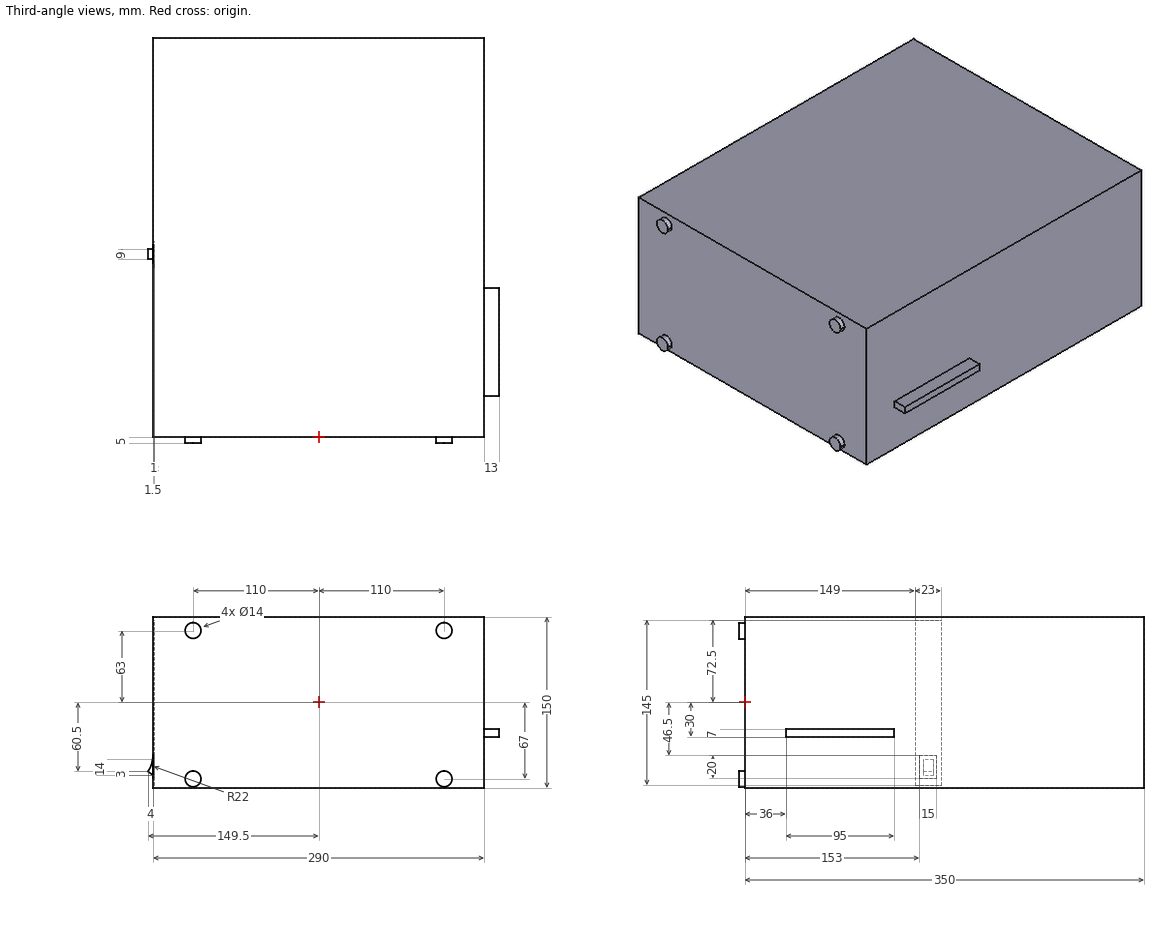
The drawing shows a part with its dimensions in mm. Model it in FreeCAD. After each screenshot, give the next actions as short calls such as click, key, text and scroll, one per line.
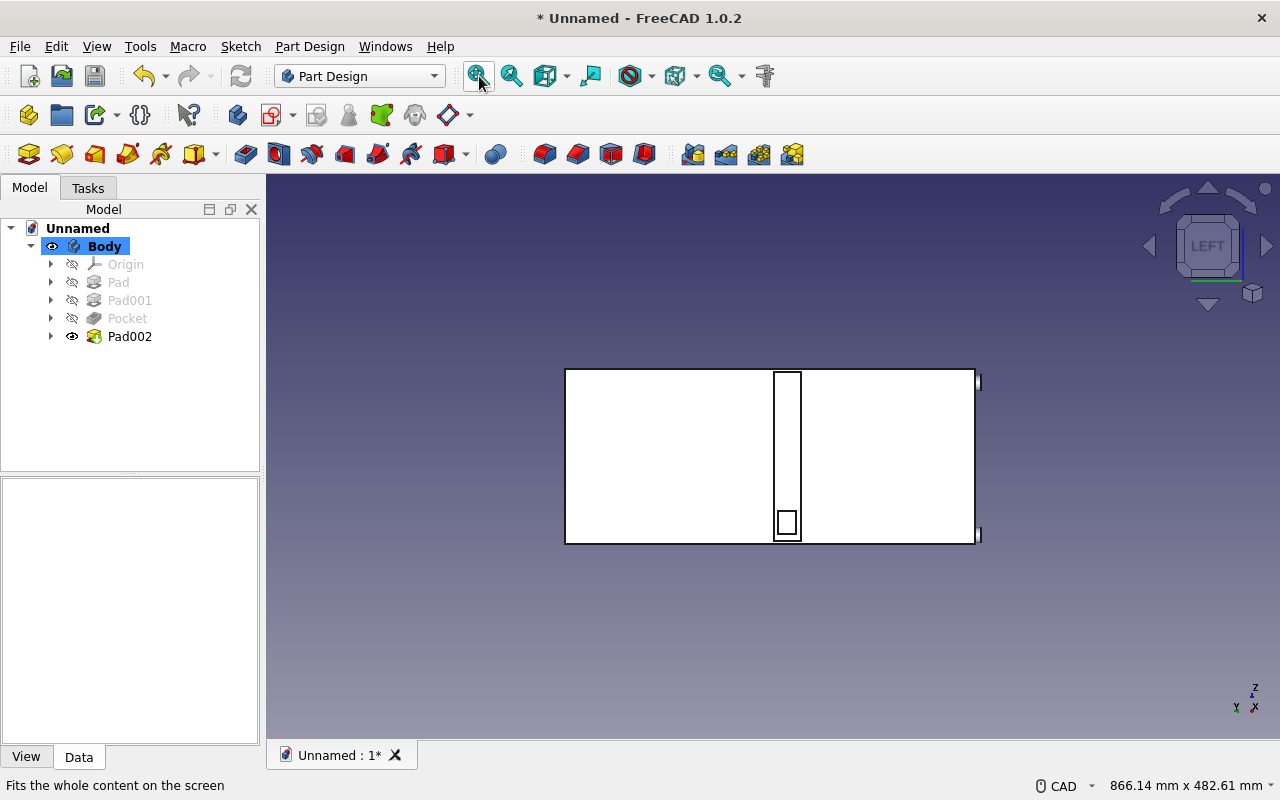
click(51, 264)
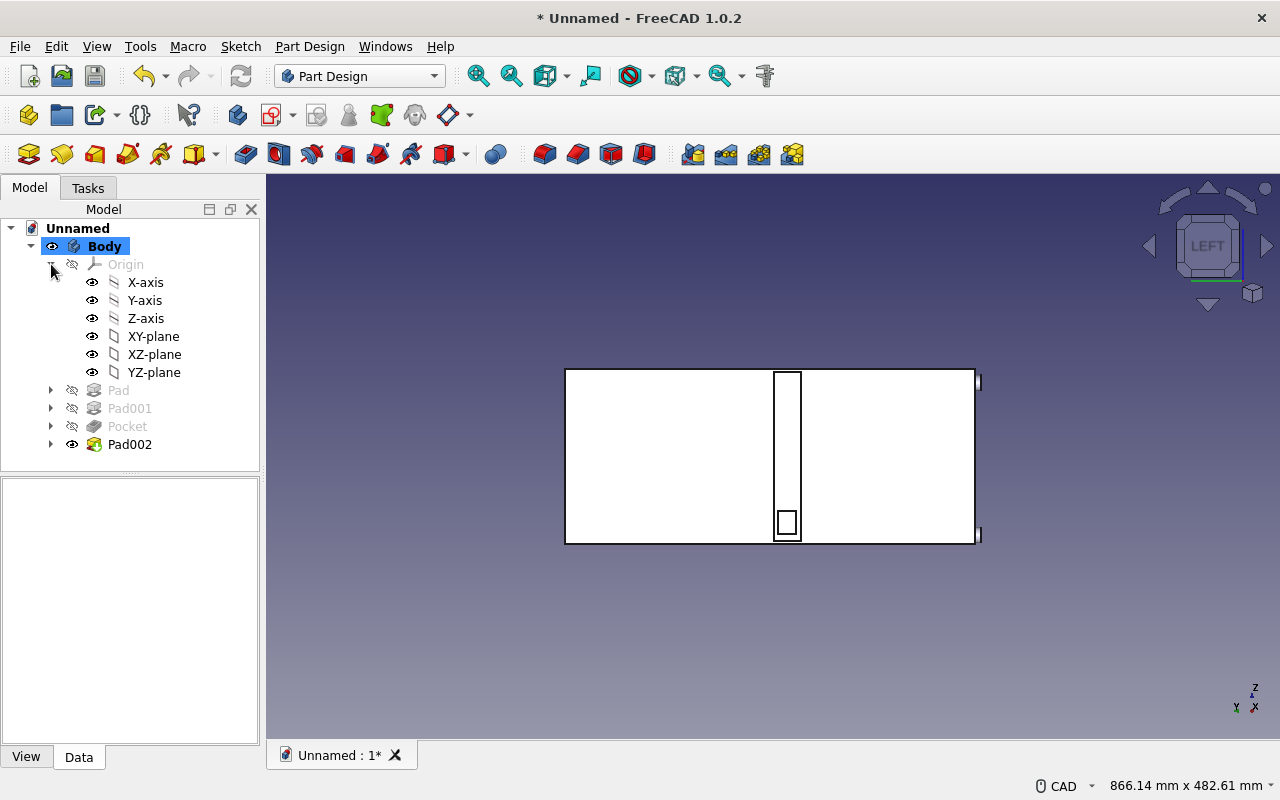
click(137, 354)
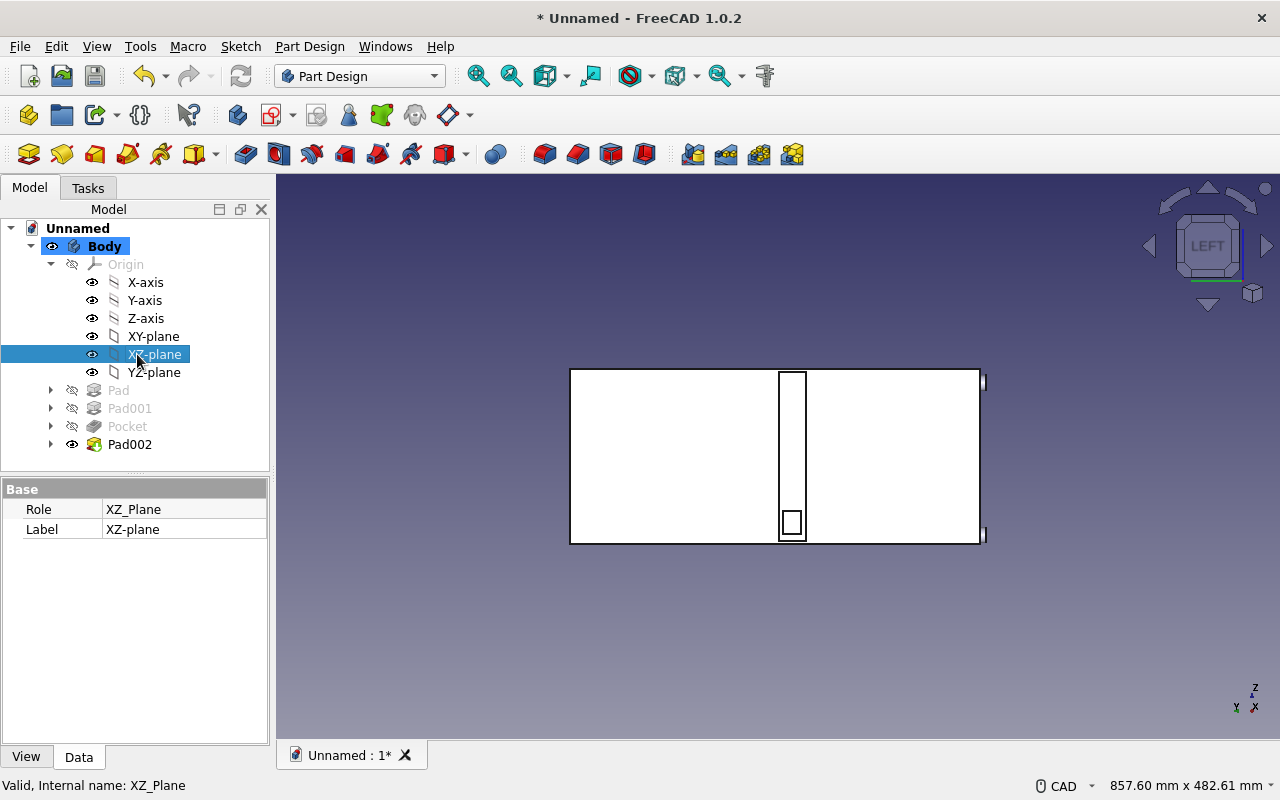
click(448, 116)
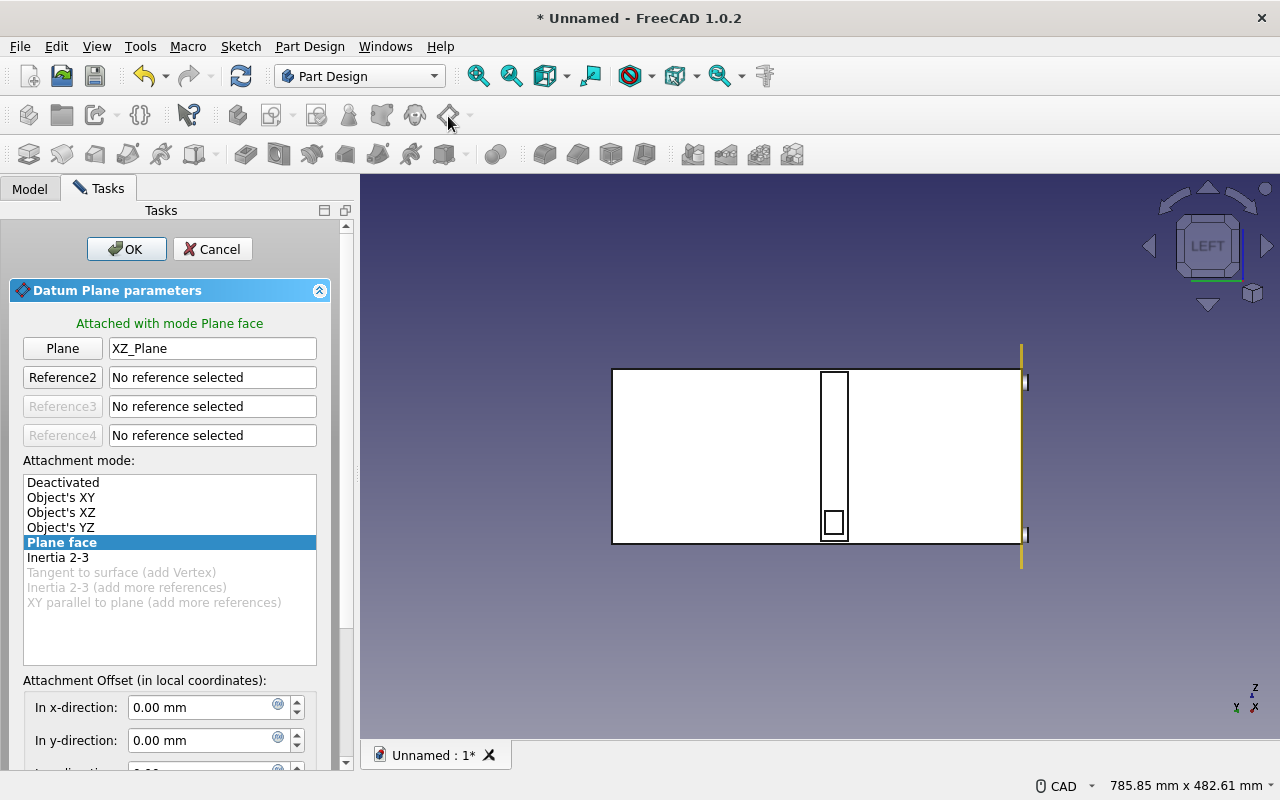
scroll(346, 495, down, 2)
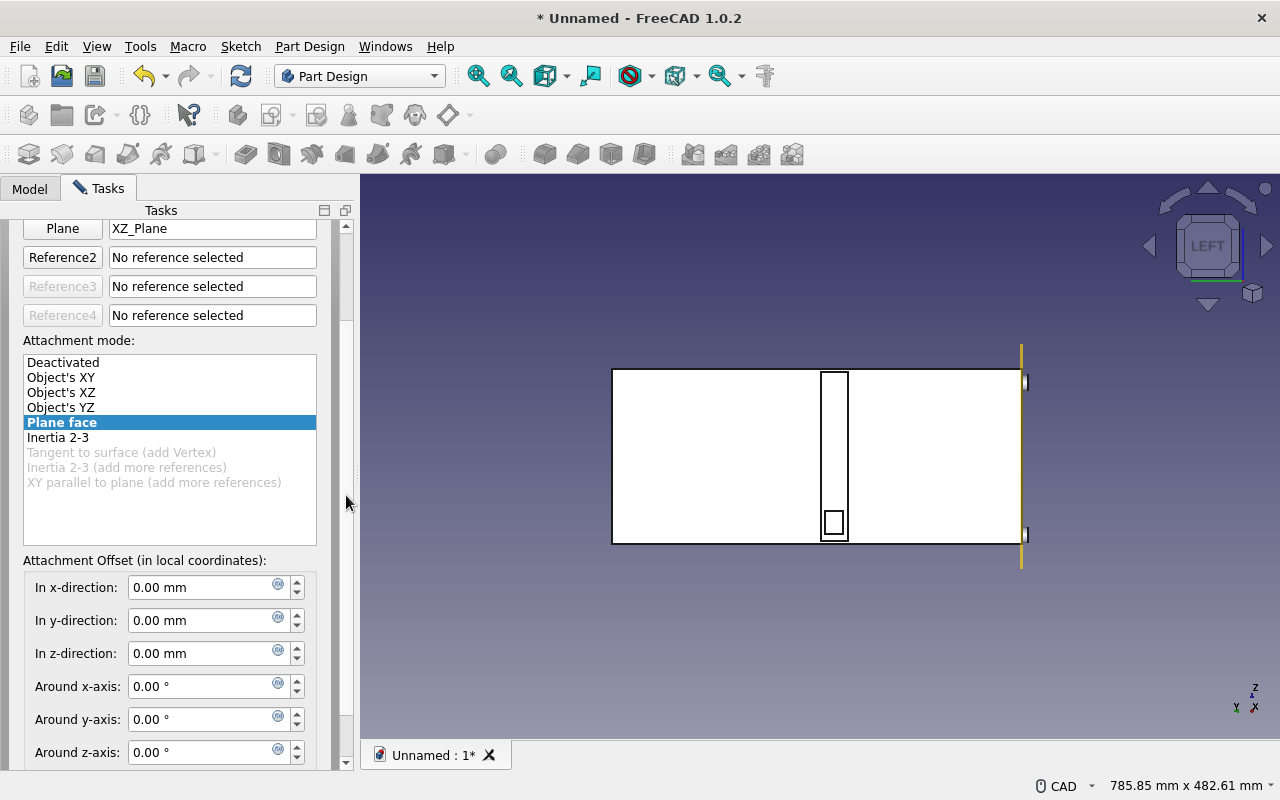
triple_click(210, 654)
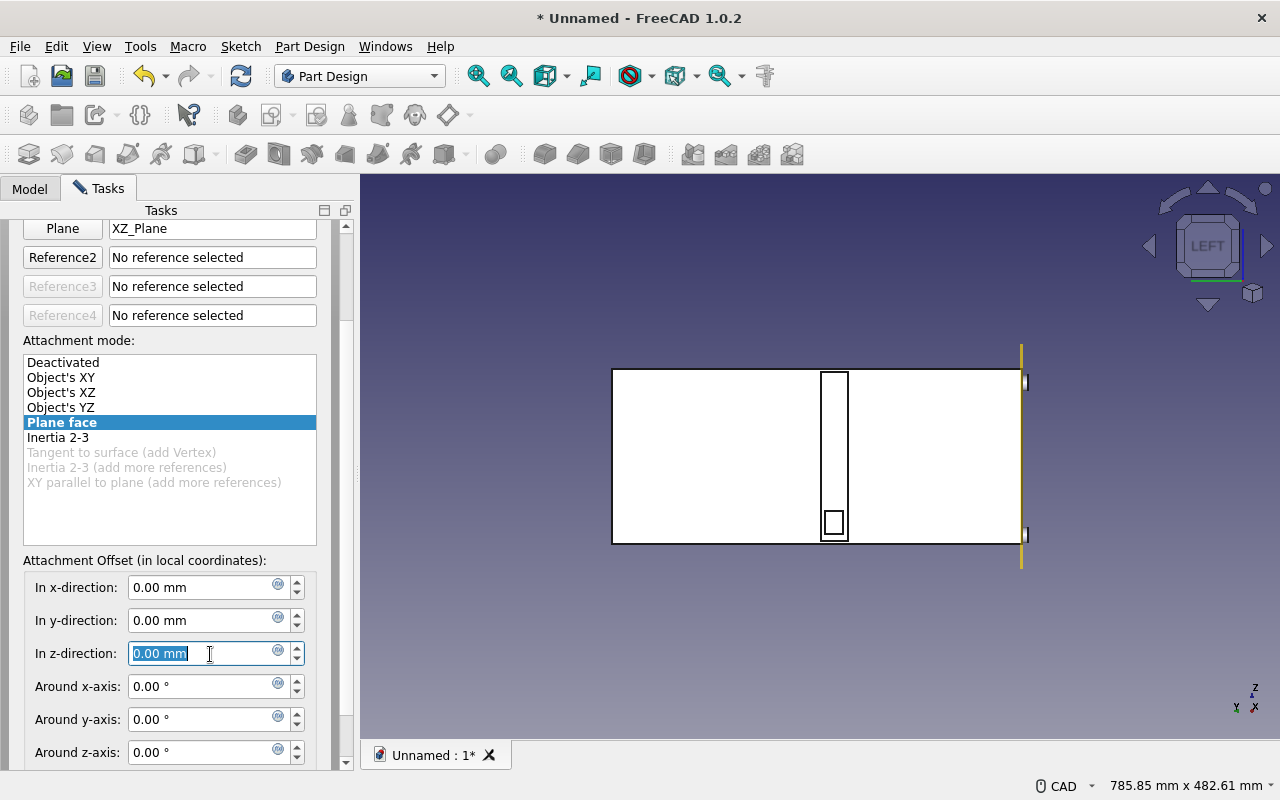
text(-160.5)
key(Tab)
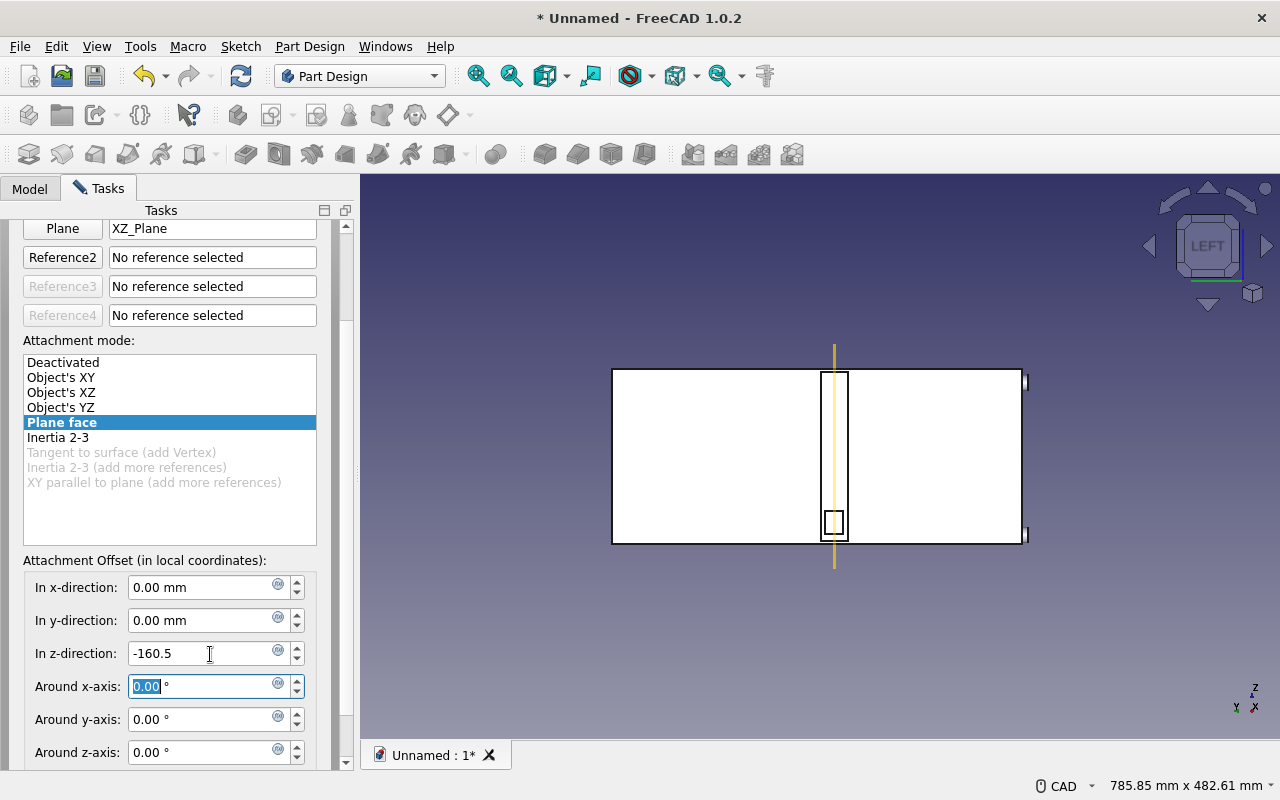
scroll(346, 495, up, 3)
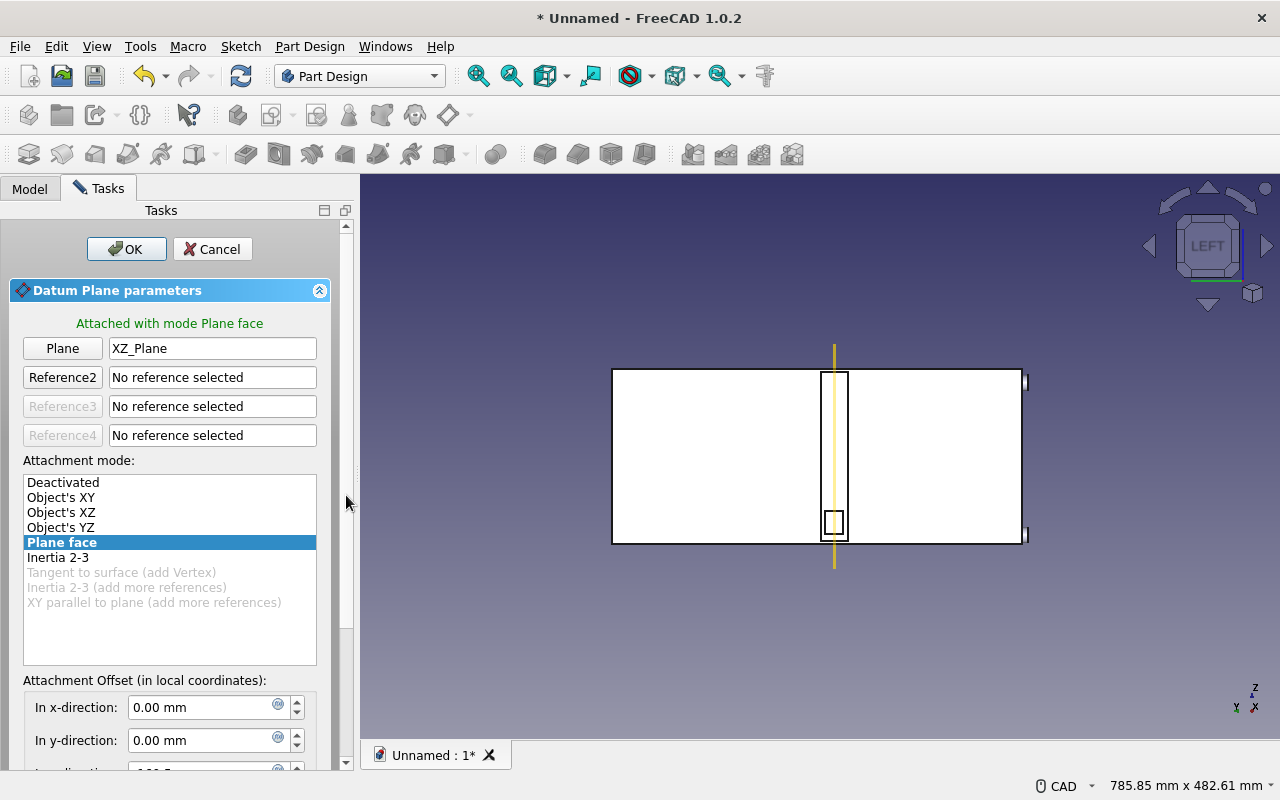
click(127, 249)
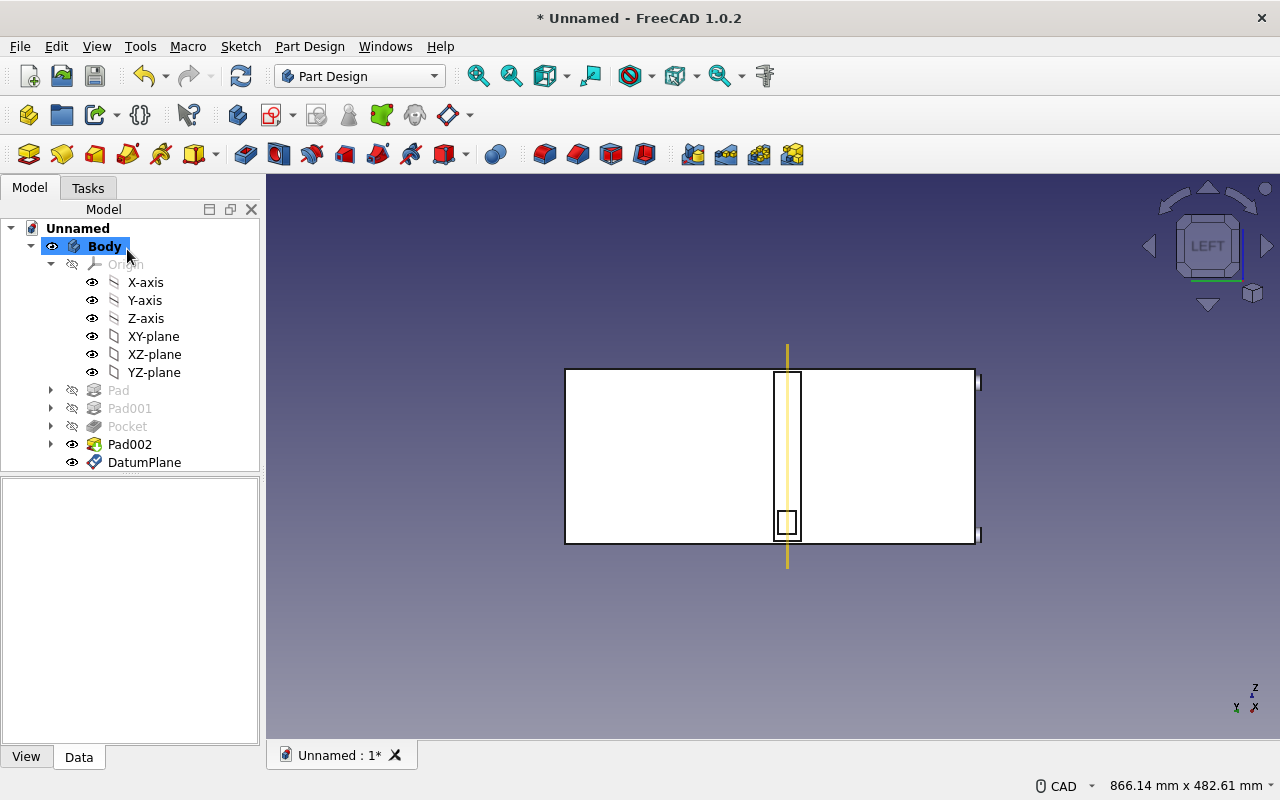
click(117, 462)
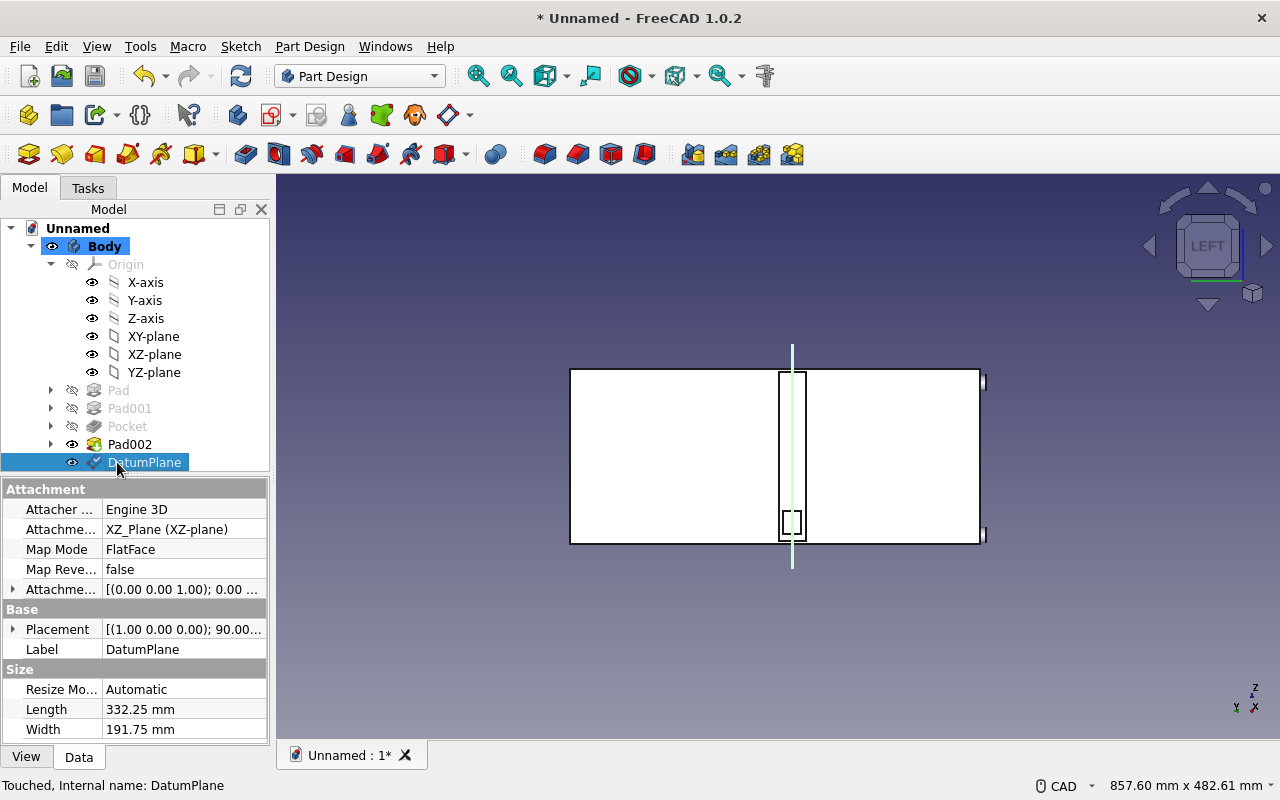
click(270, 116)